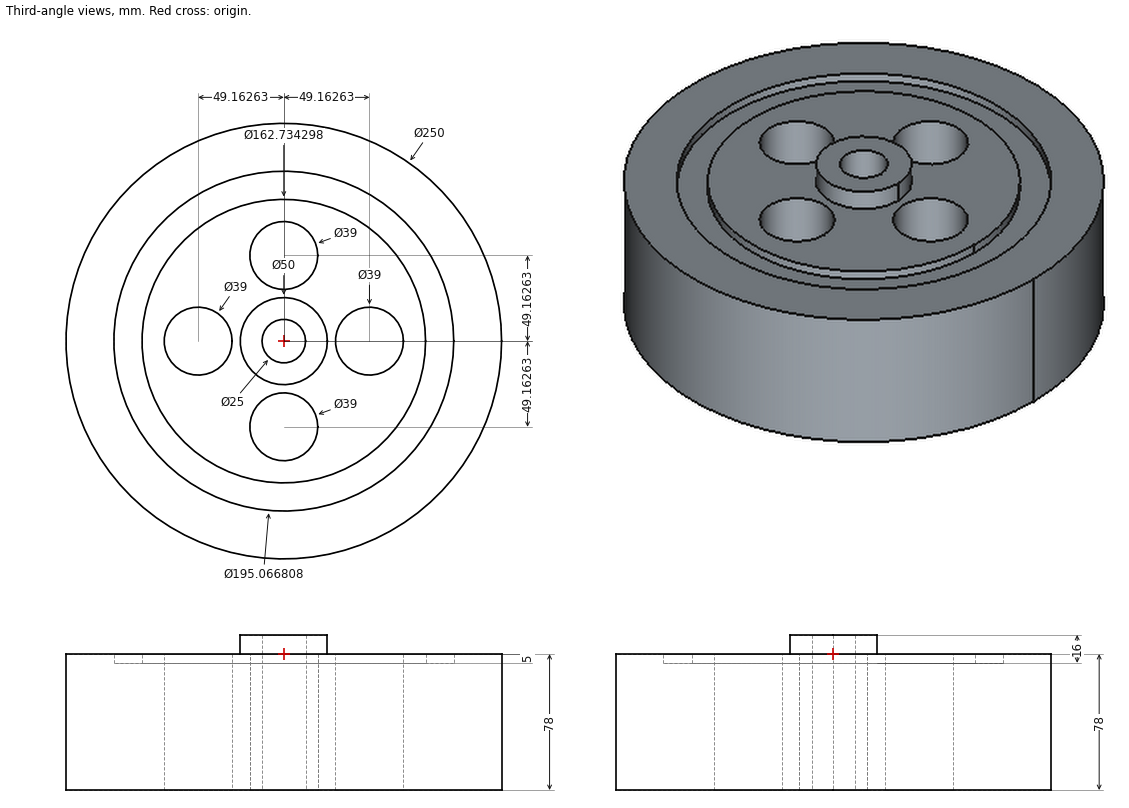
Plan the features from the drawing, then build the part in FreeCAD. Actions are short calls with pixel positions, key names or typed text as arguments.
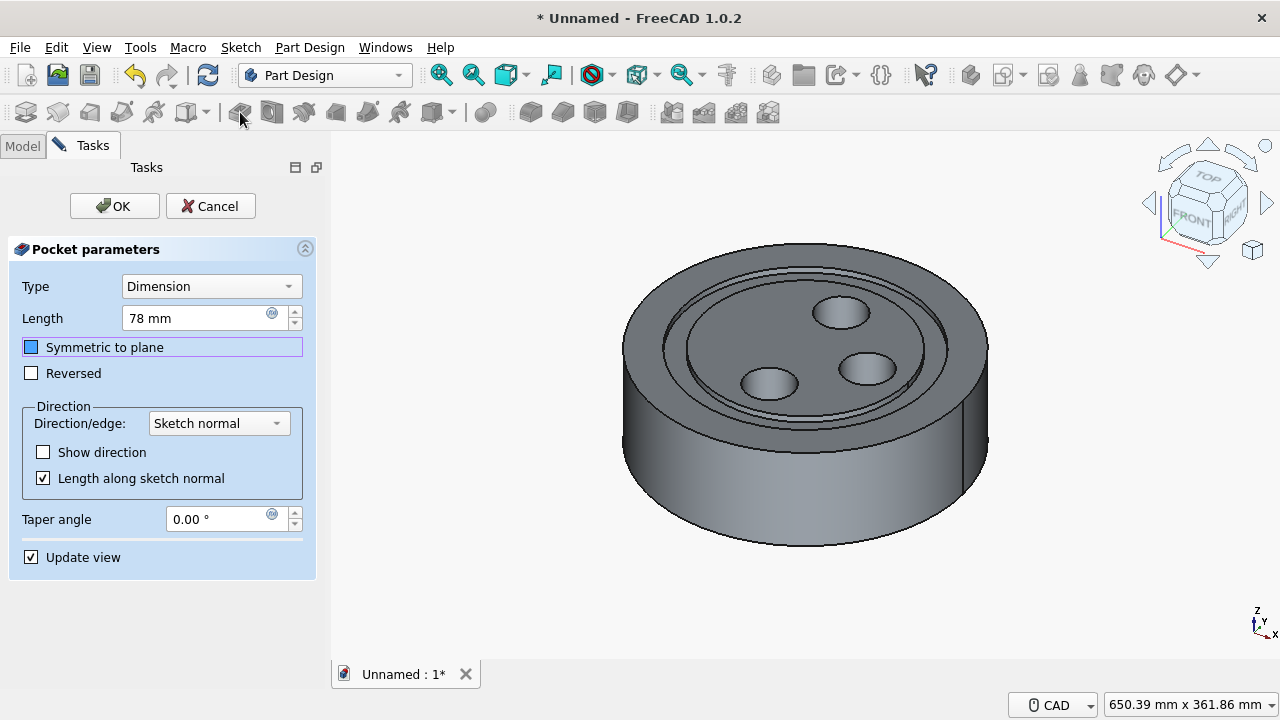
click(115, 206)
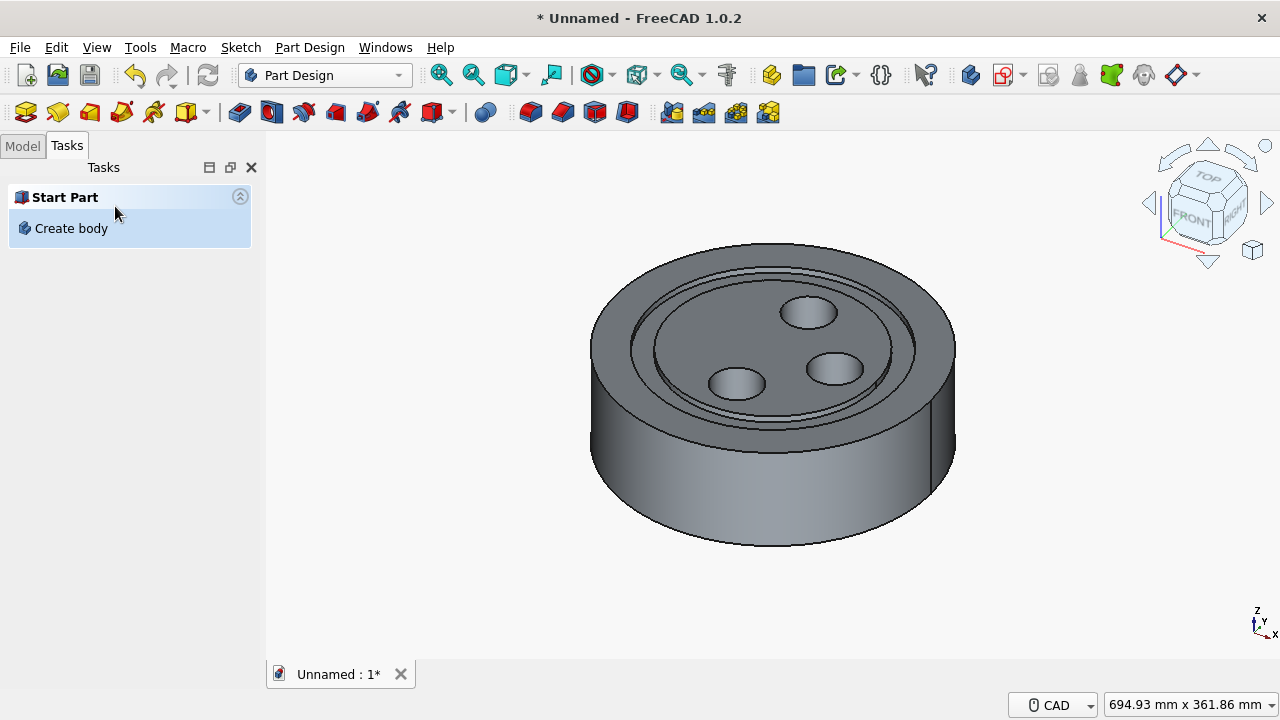
click(1004, 76)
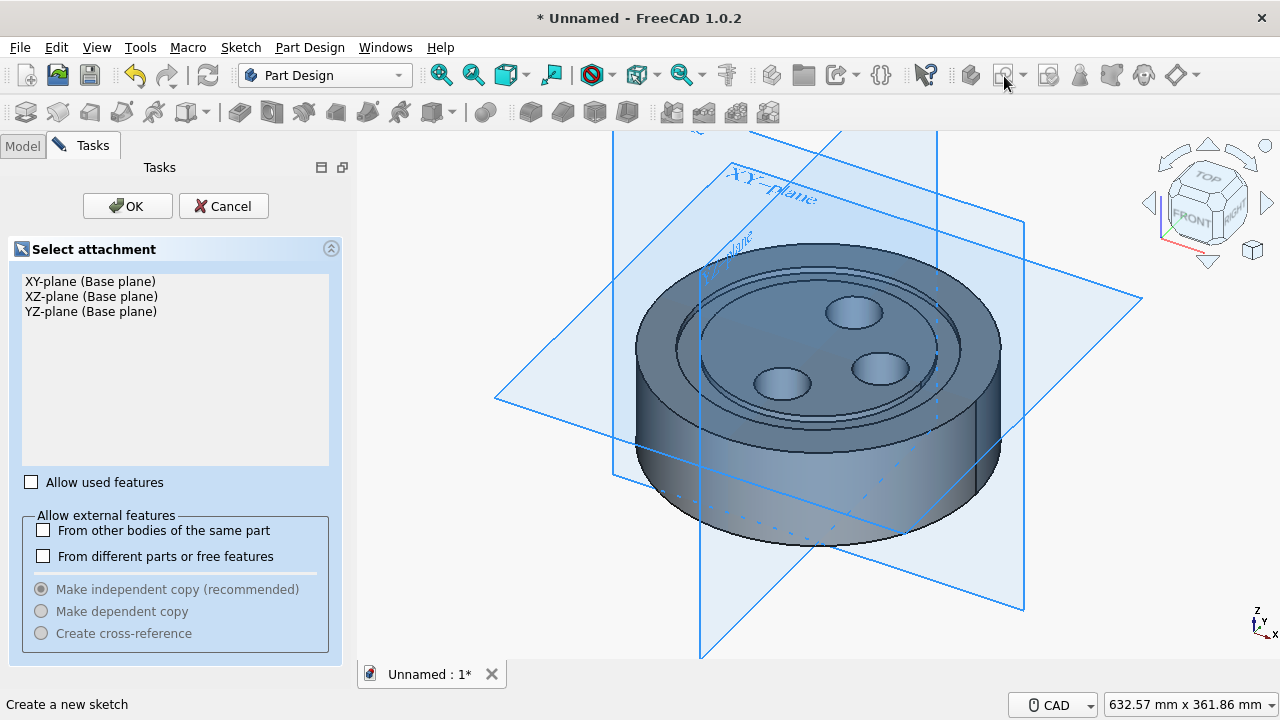
click(82, 282)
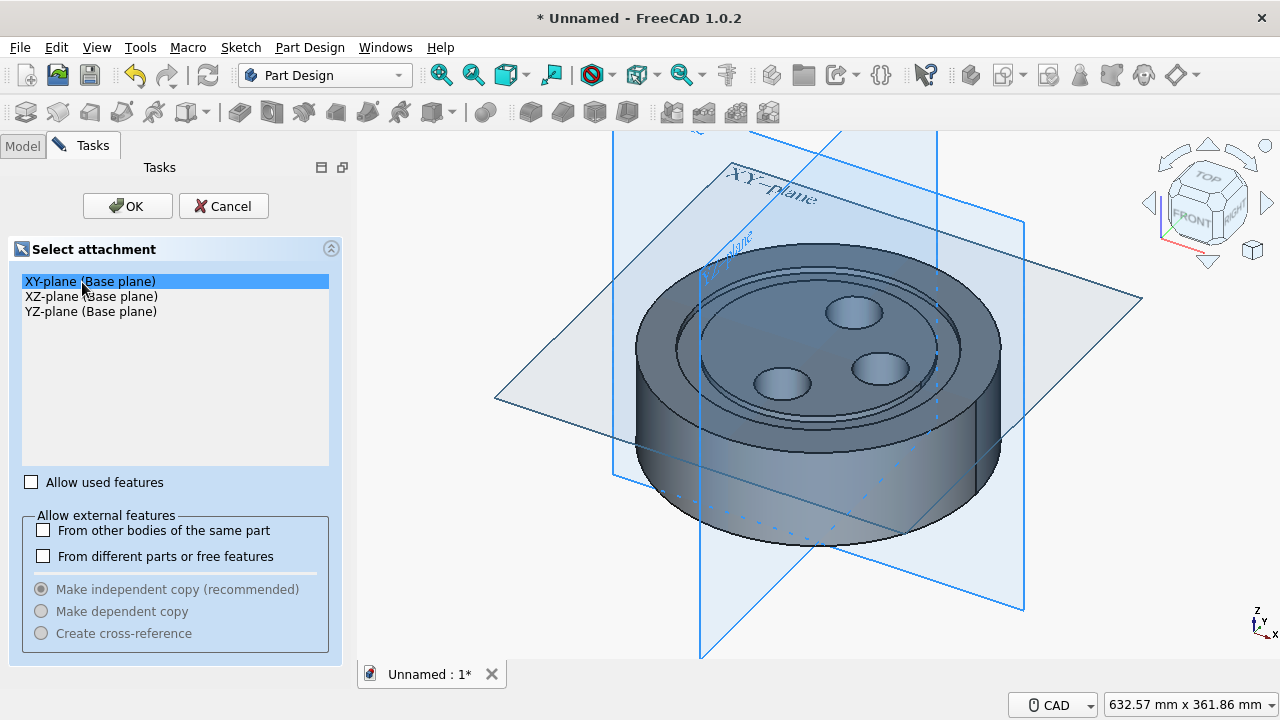
click(128, 206)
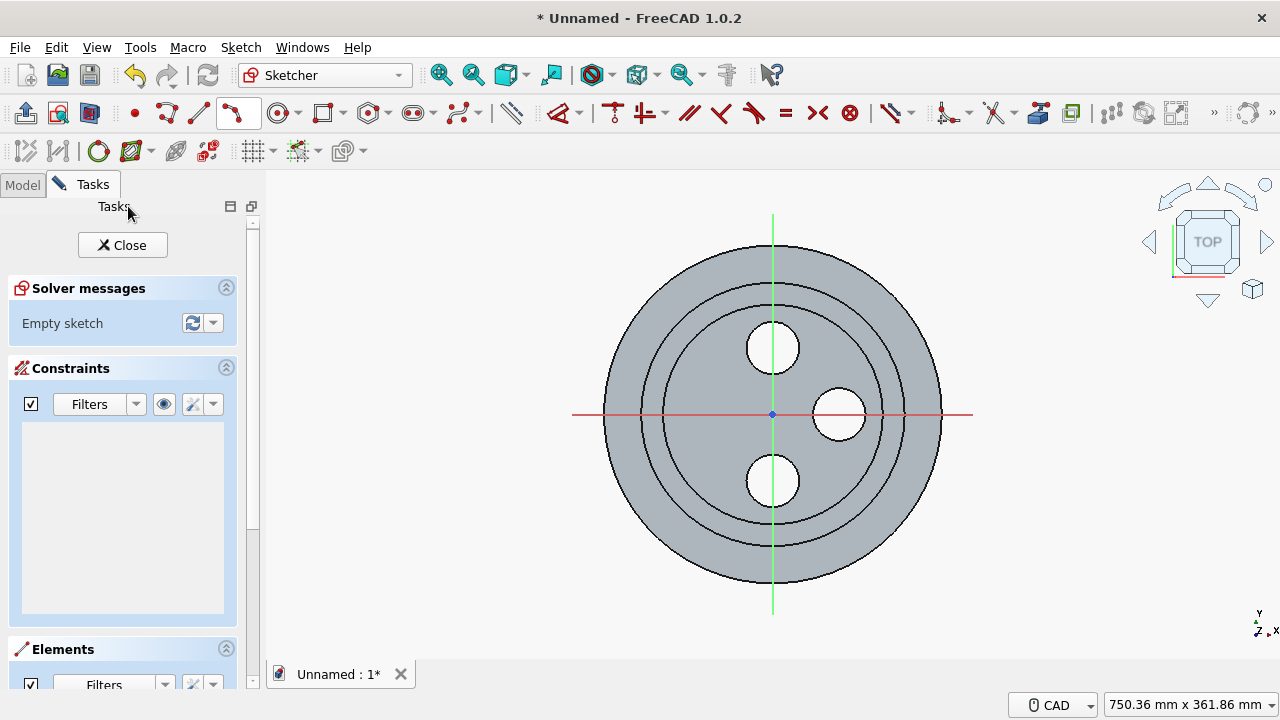
scroll(731, 414, up, 9)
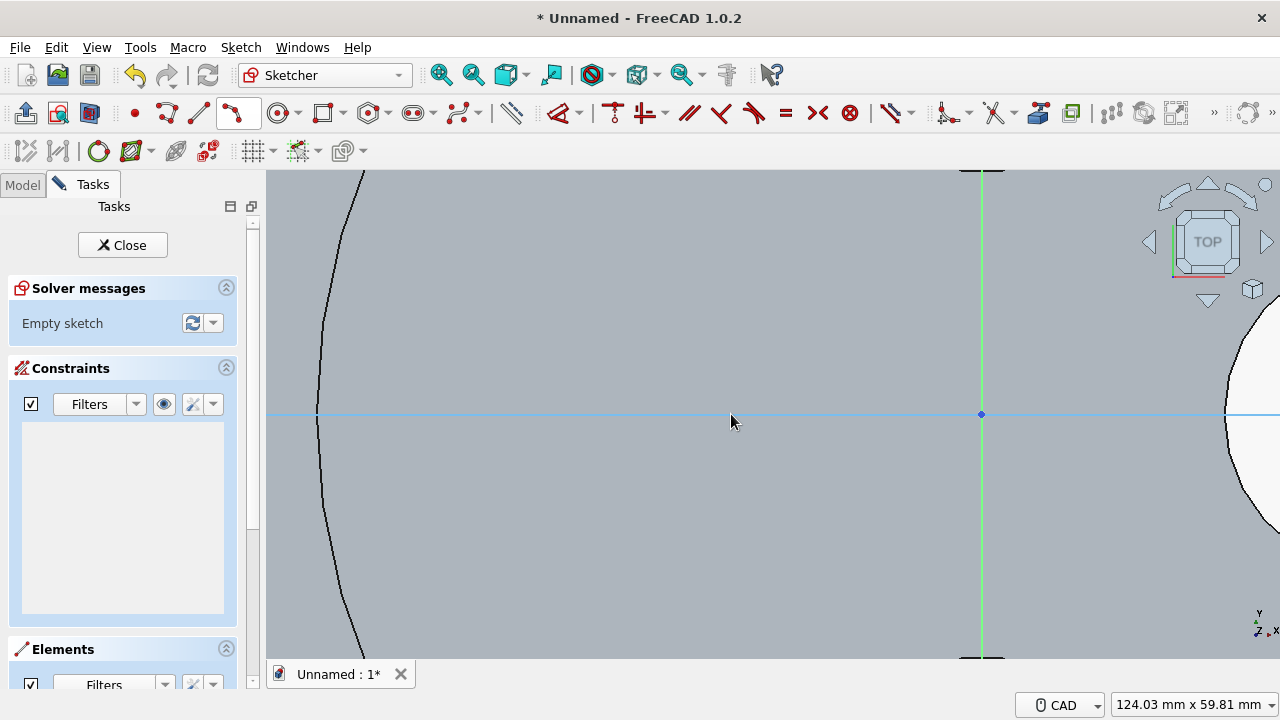
click(278, 114)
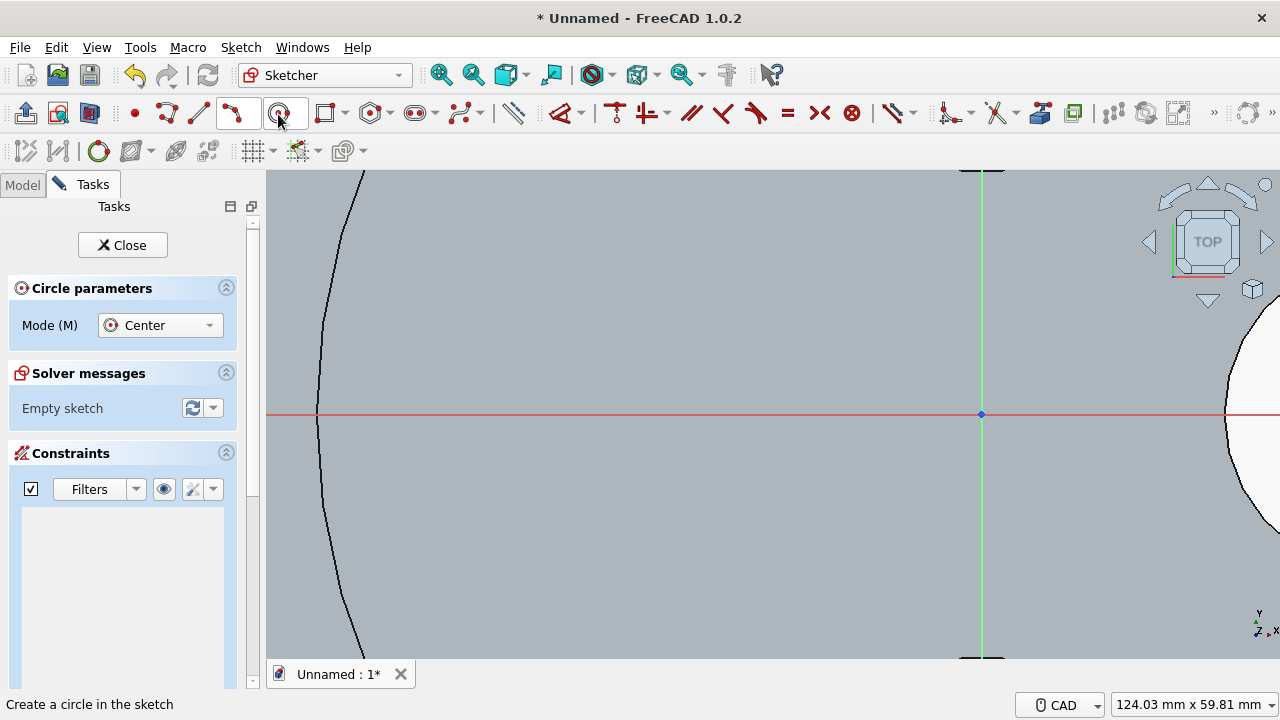
click(580, 414)
move(693, 302)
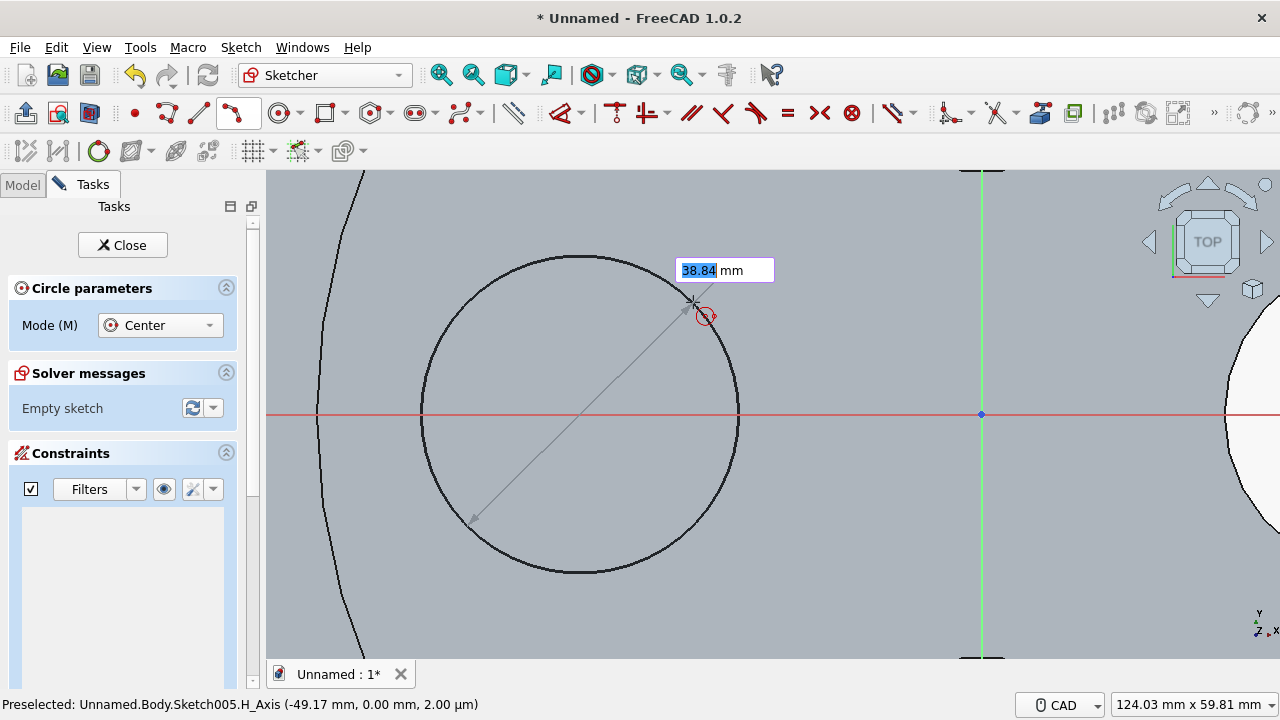
text(39)
key(Return)
key(Escape)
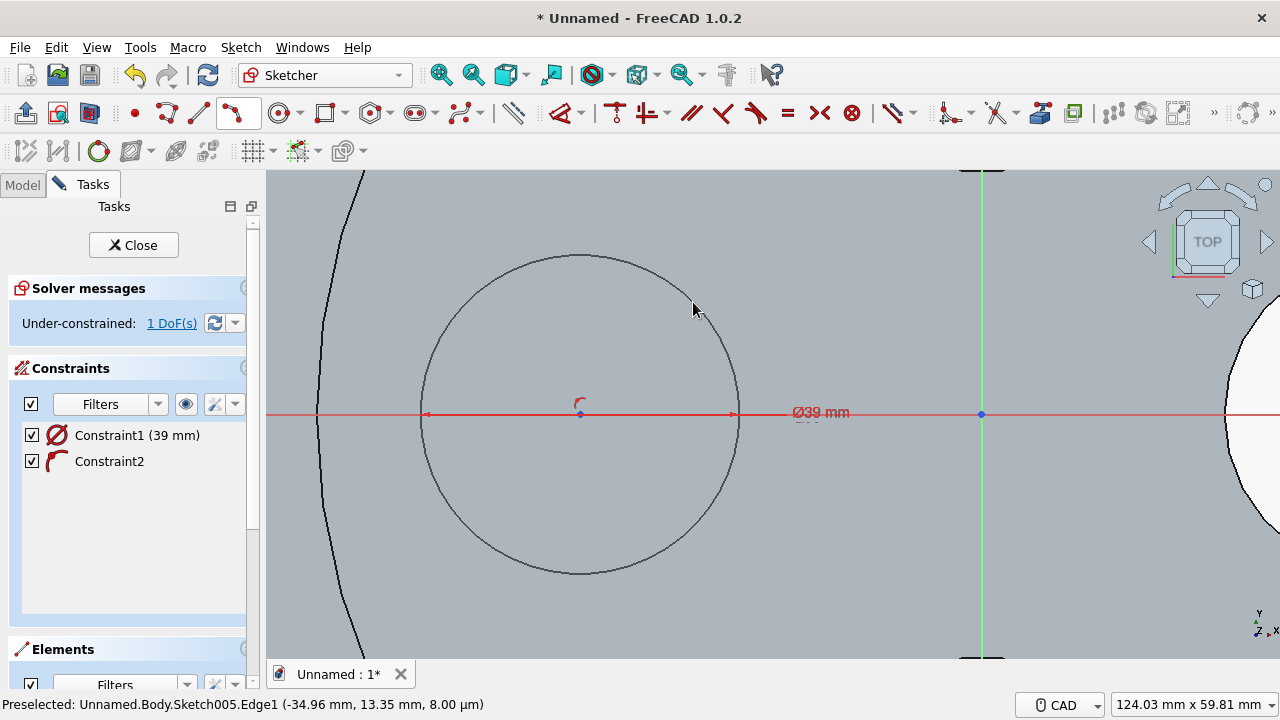
click(560, 114)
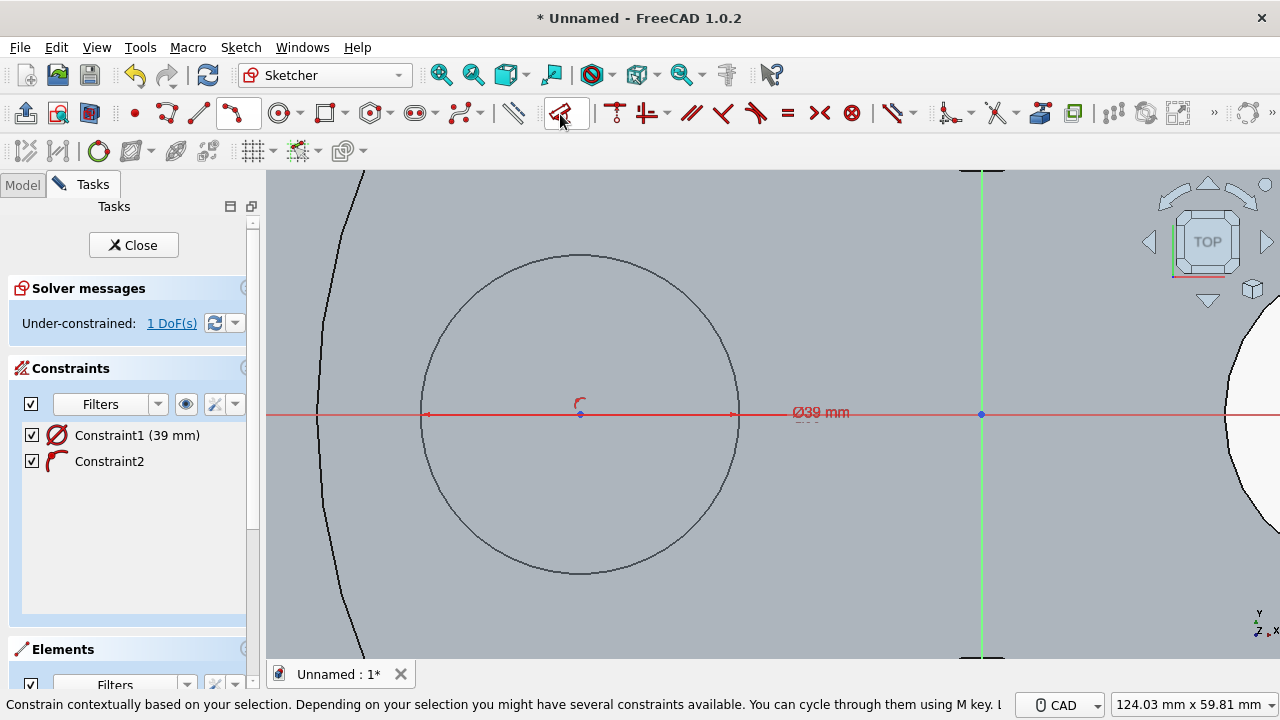
click(580, 414)
click(781, 448)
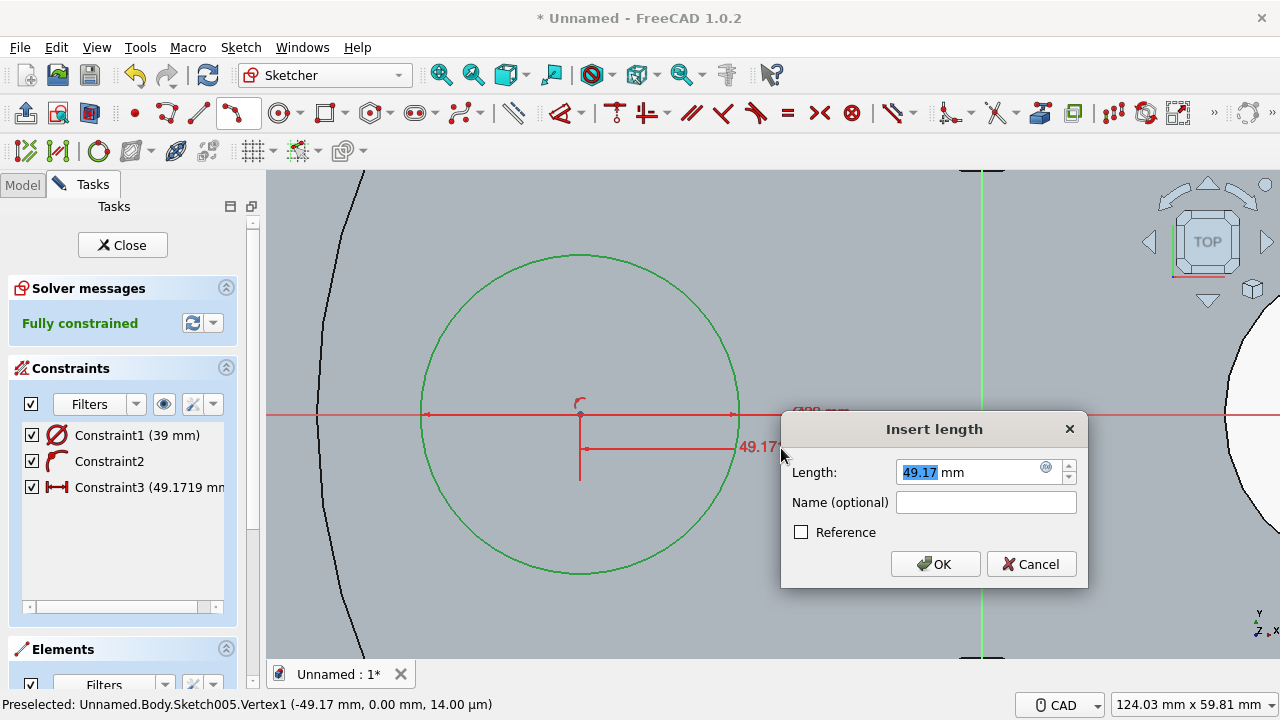
text(49.16263)
key(Return)
key(Escape)